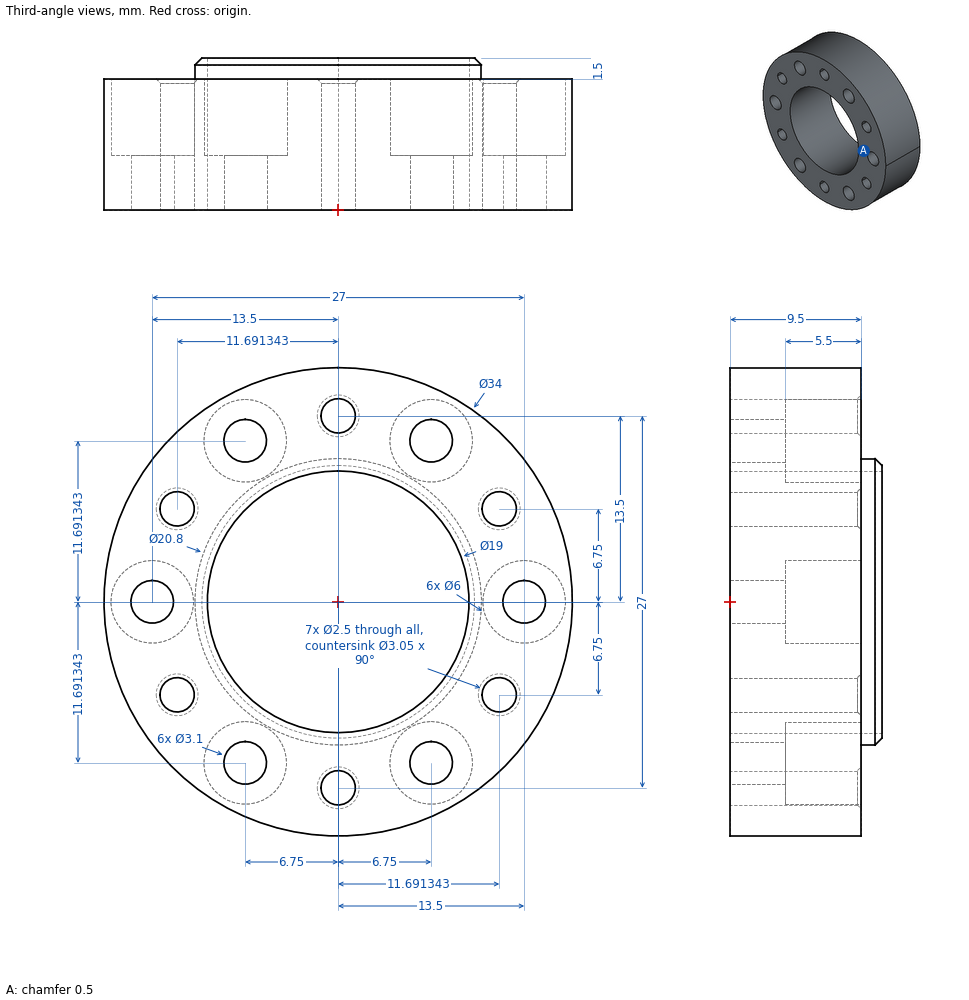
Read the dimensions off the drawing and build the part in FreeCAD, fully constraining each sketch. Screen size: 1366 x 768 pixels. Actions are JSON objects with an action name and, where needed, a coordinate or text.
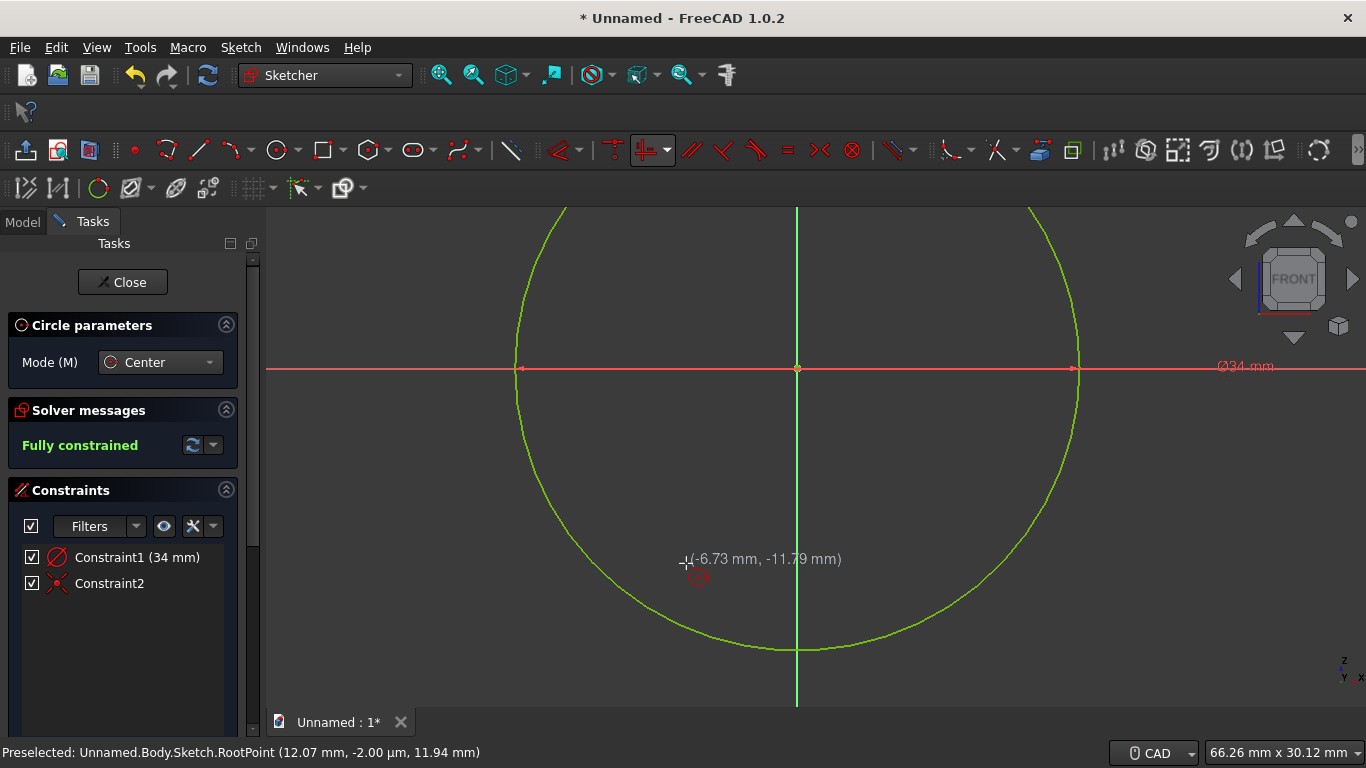
{"action": "left_click", "coordinate": [685, 563]}
{"action": "mouse_move", "coordinate": [704, 544]}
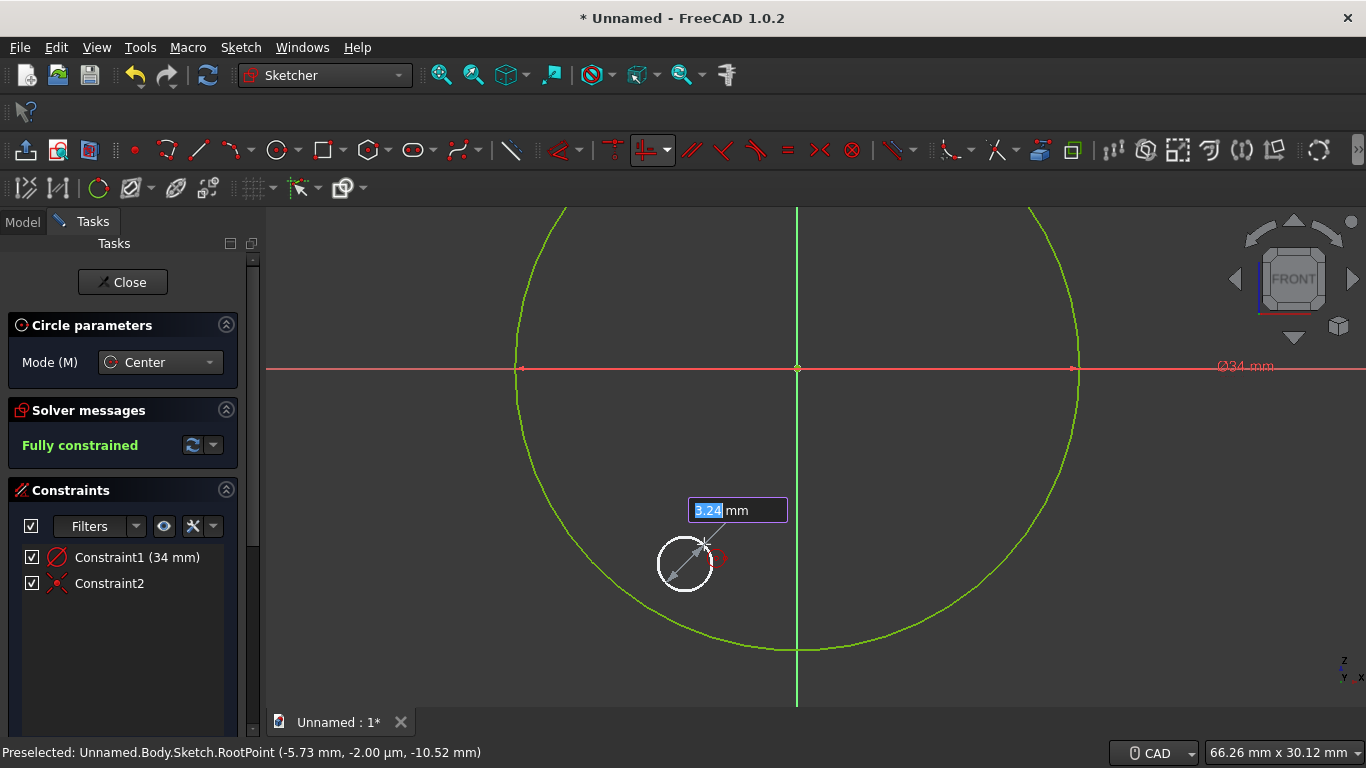
{"action": "type", "text": "3.1"}
{"action": "key", "text": "Return"}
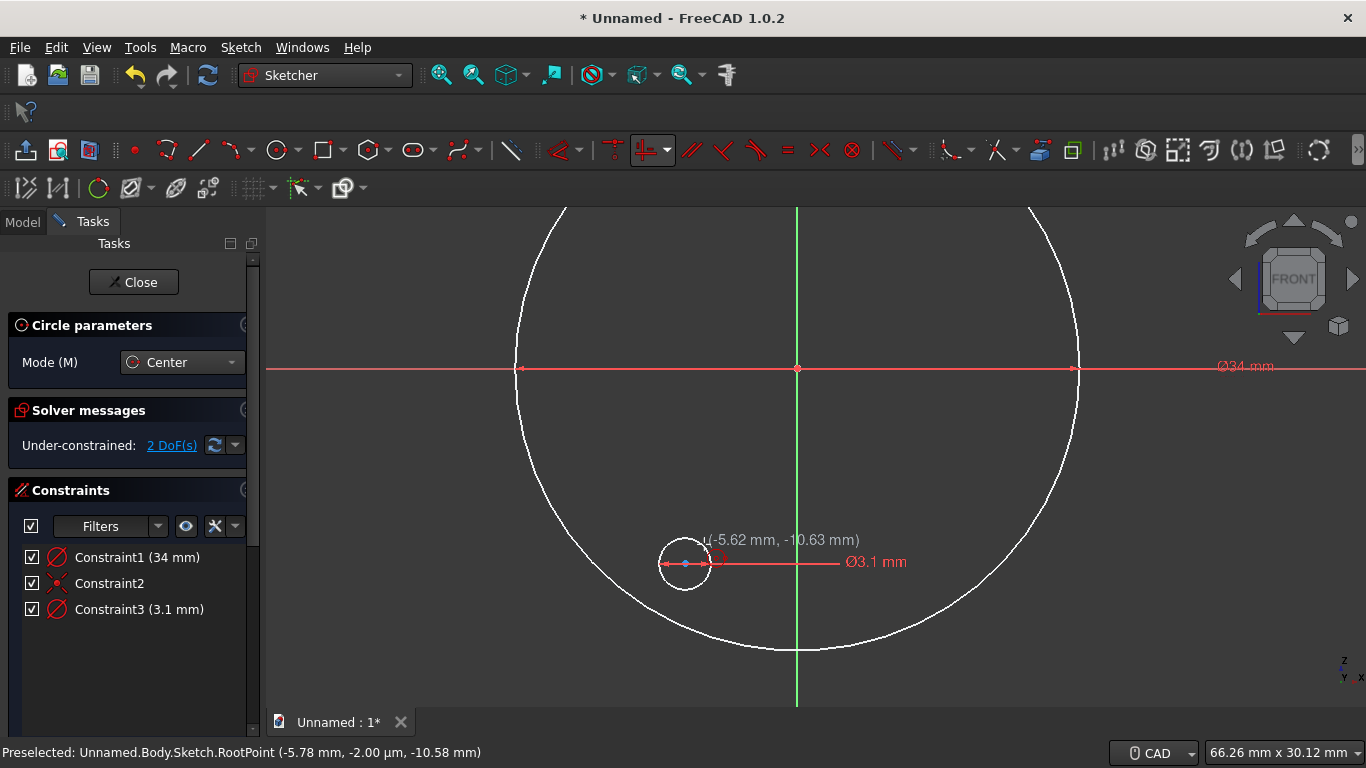
{"action": "left_click", "coordinate": [573, 369]}
{"action": "mouse_move", "coordinate": [591, 350]}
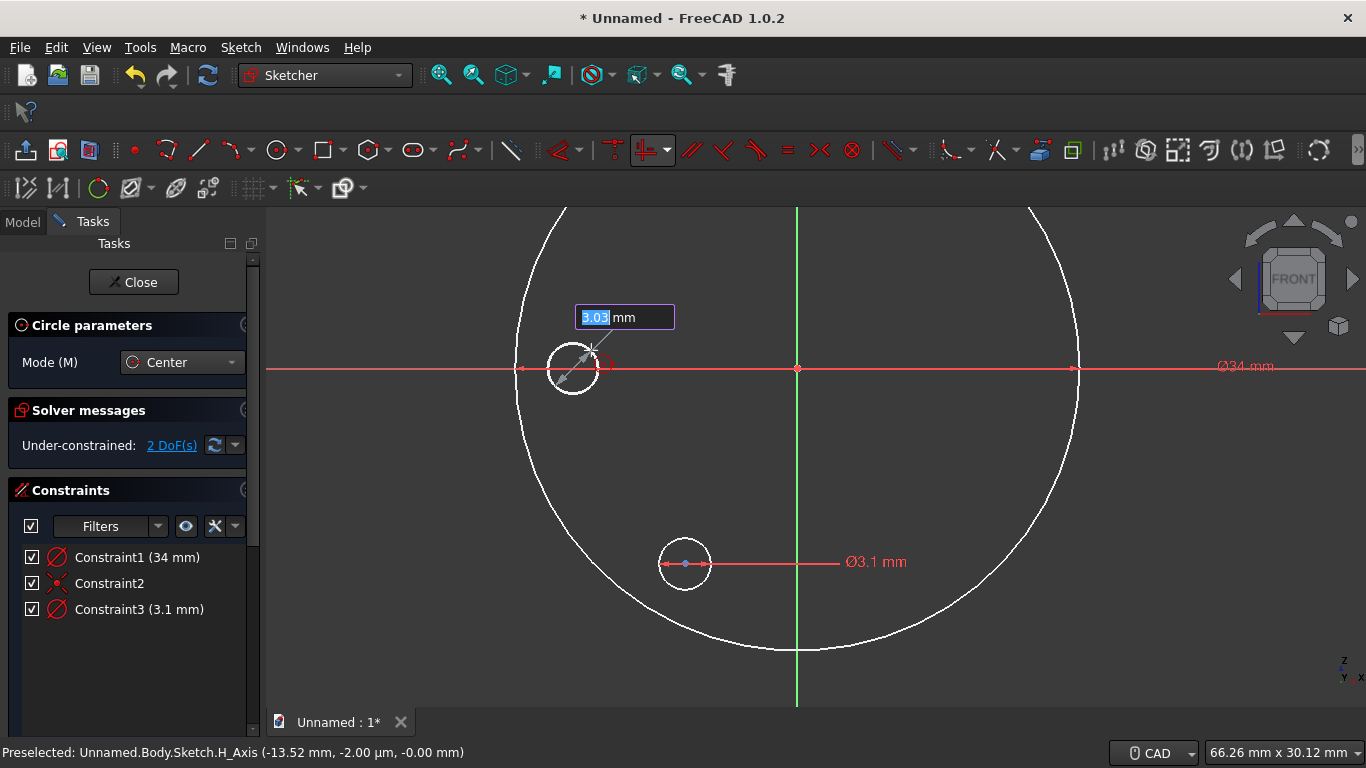
{"action": "type", "text": "3.1"}
{"action": "key", "text": "Return"}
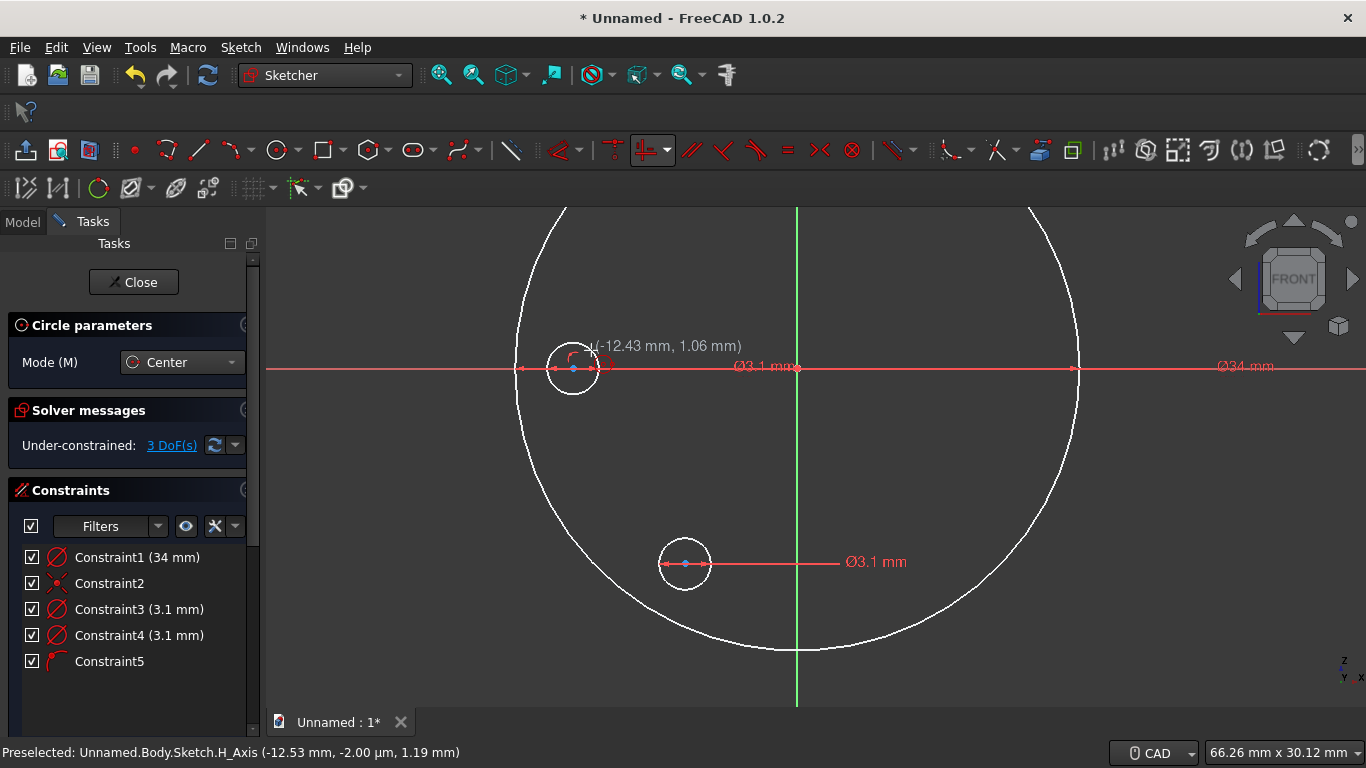
{"action": "left_click", "coordinate": [797, 369]}
{"action": "mouse_move", "coordinate": [909, 257]}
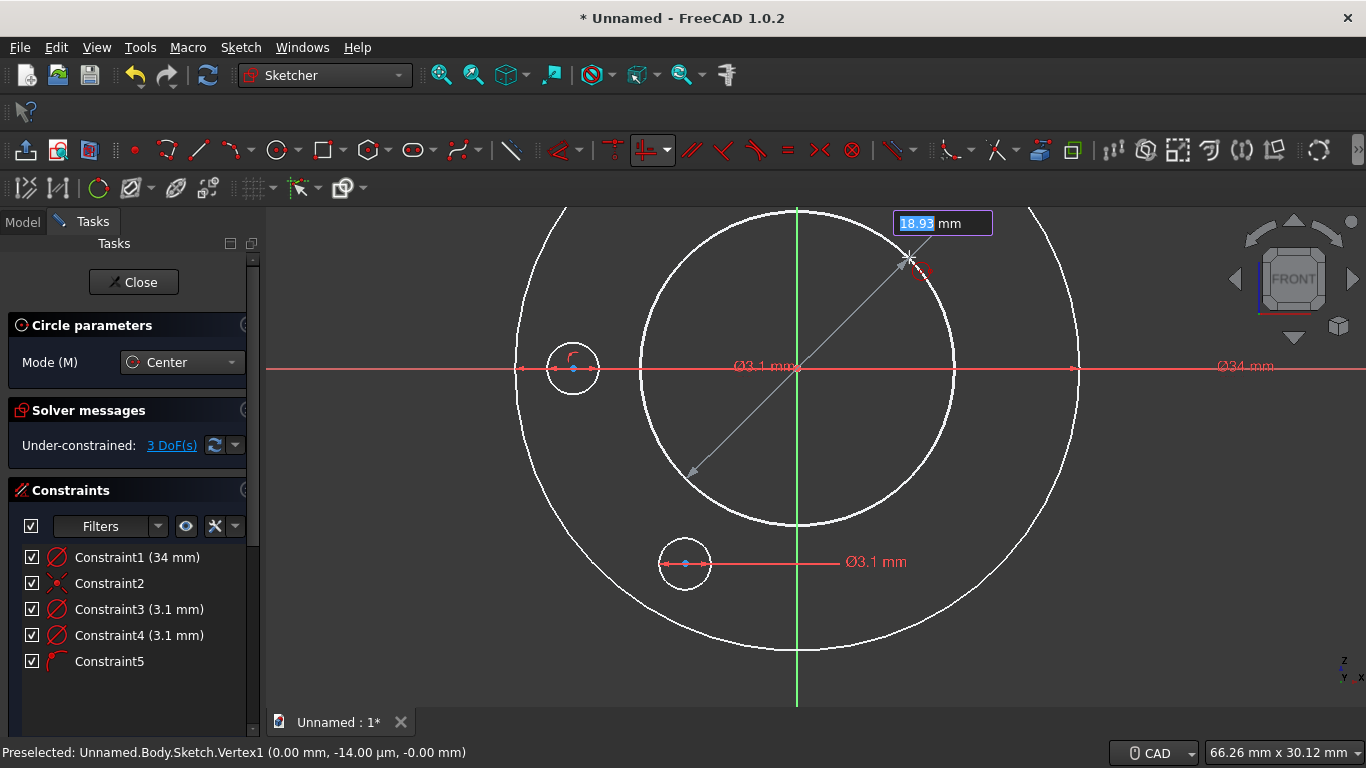
{"action": "type", "text": "19"}
{"action": "key", "text": "Return"}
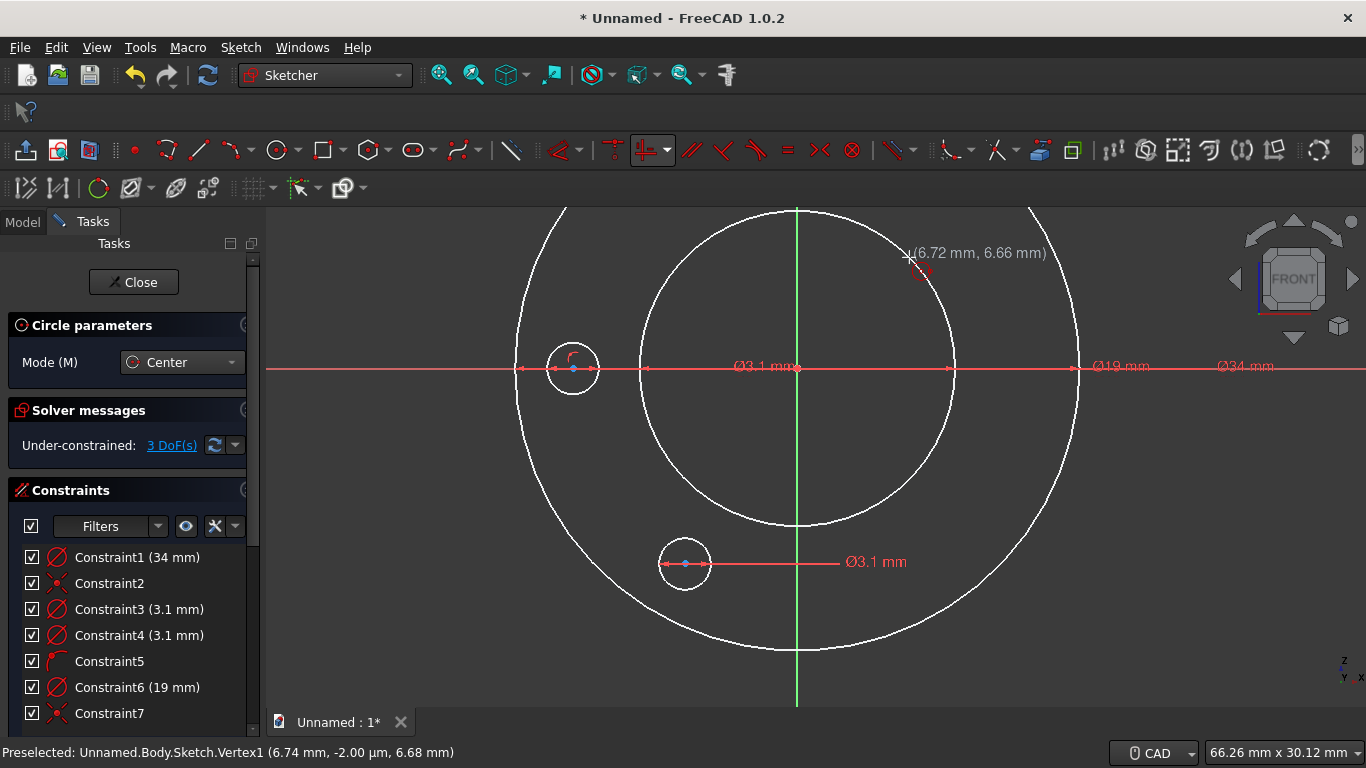
{"action": "scroll", "coordinate": [687, 565], "scroll_direction": "down", "scroll_amount": 3}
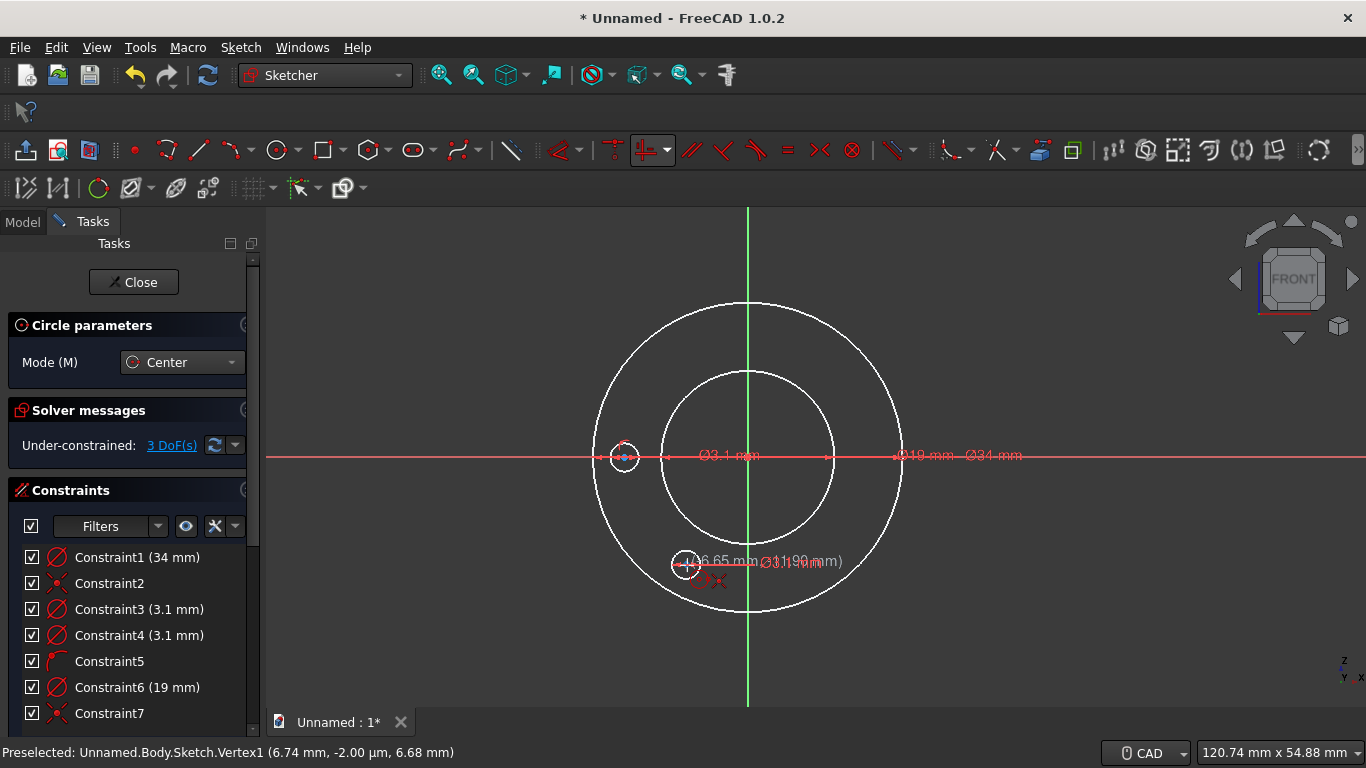
{"action": "scroll", "coordinate": [686, 351], "scroll_direction": "up", "scroll_amount": 3}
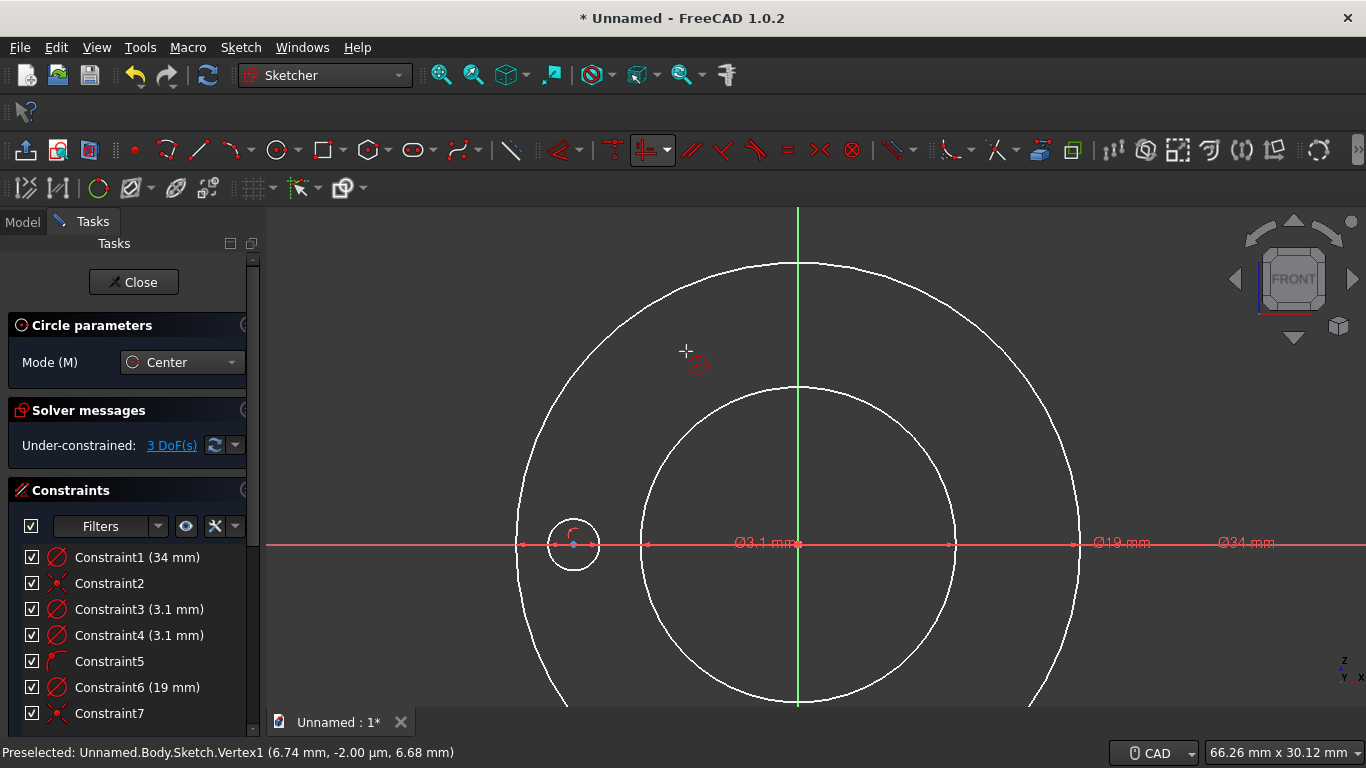
{"action": "left_click", "coordinate": [686, 351]}
{"action": "mouse_move", "coordinate": [704, 333]}